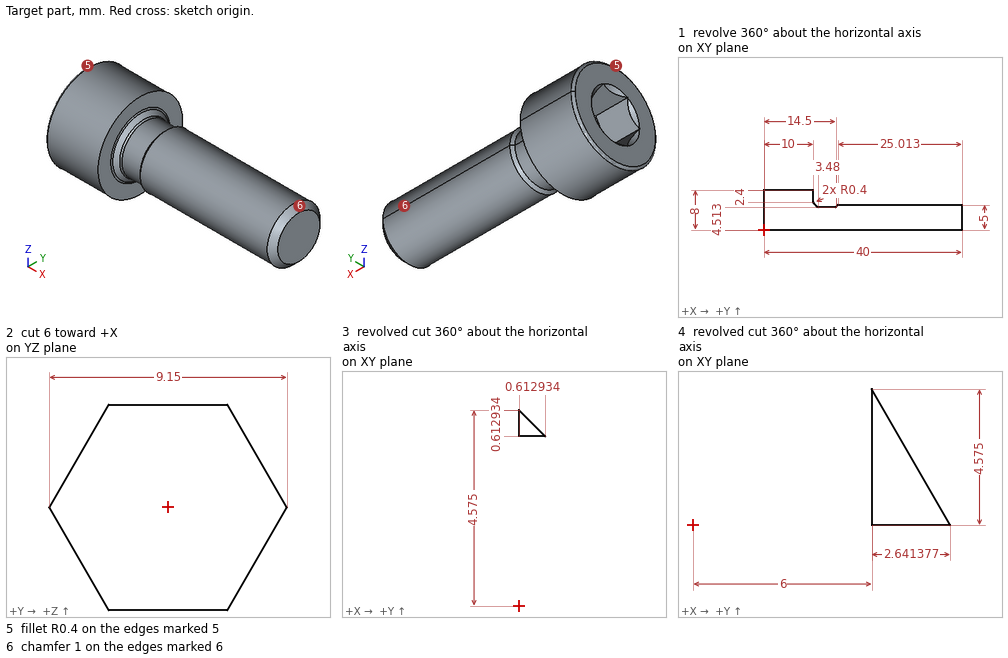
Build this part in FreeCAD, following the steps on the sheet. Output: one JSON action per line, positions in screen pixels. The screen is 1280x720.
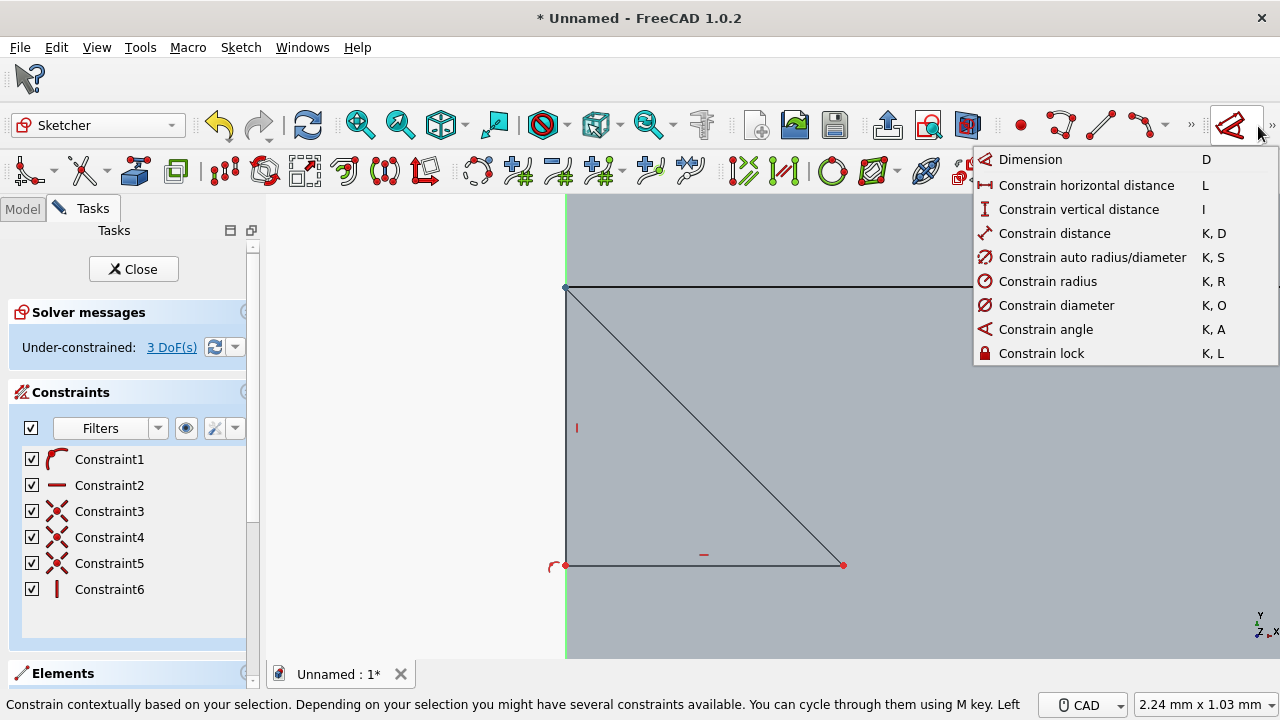
{"action": "left_click", "coordinate": [1126, 209]}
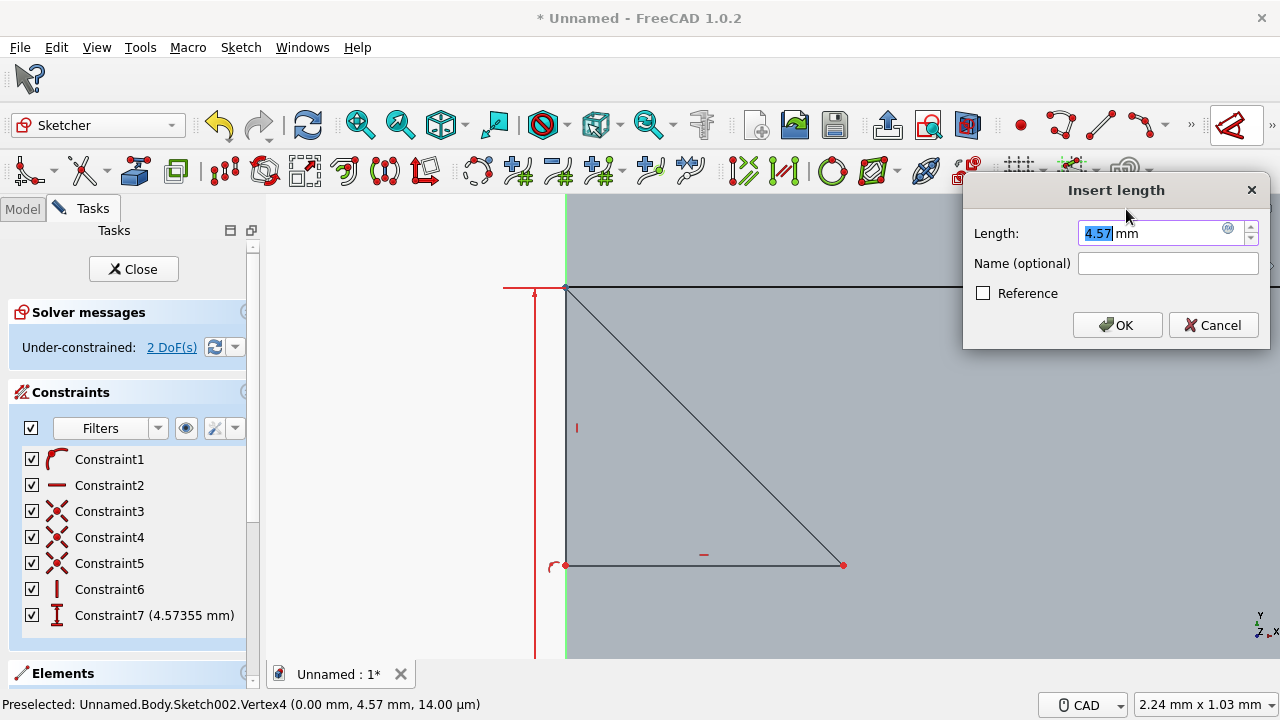
{"action": "type", "text": "4.575"}
{"action": "key", "text": "Return"}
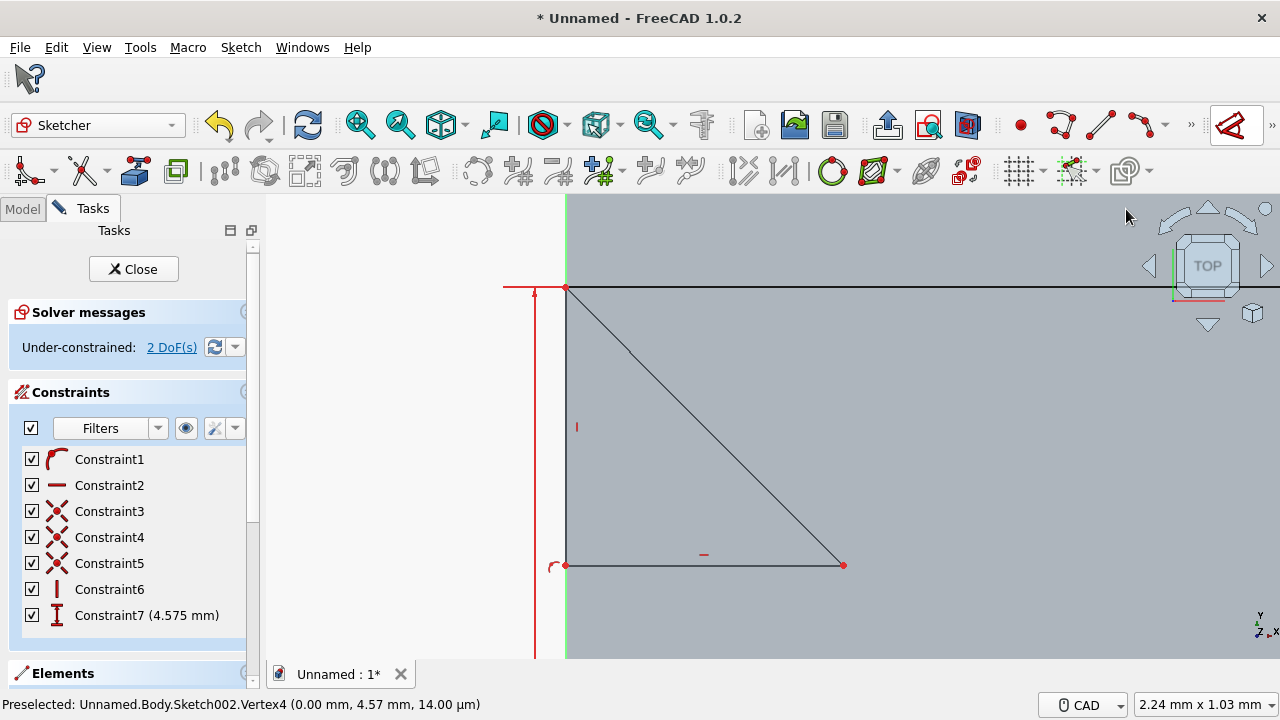
{"action": "left_click", "coordinate": [649, 566]}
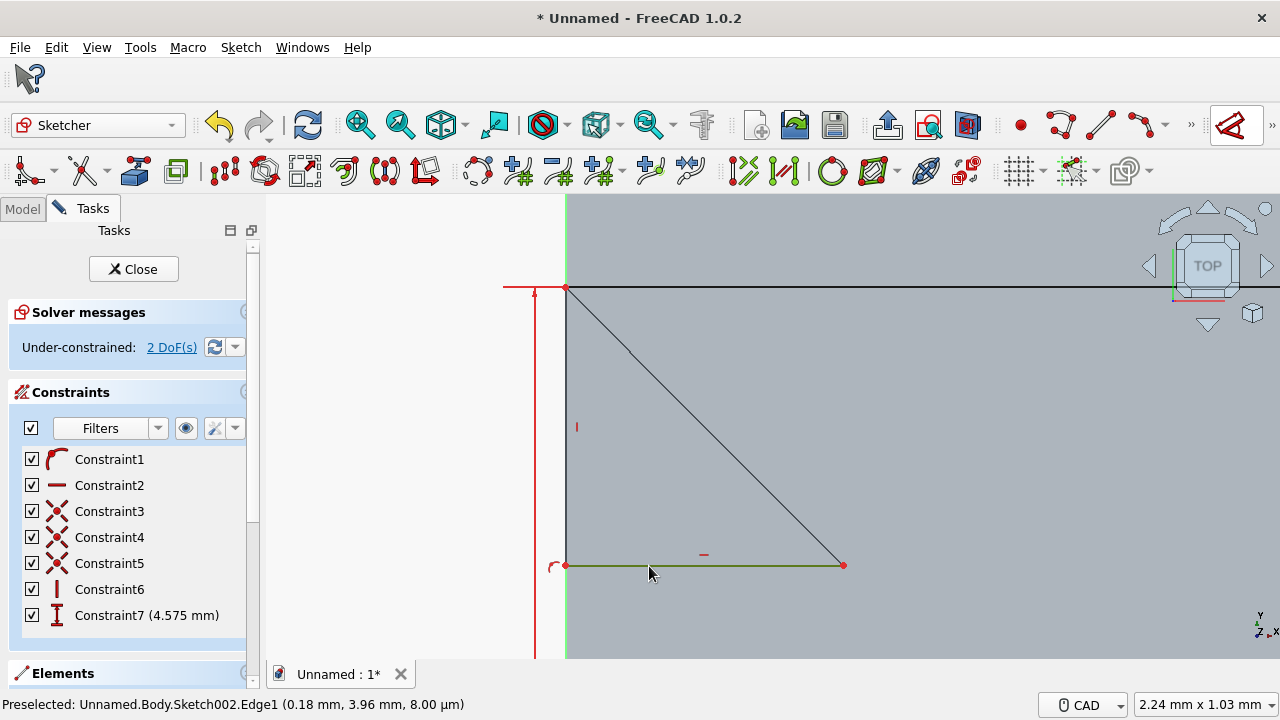
{"action": "left_click", "coordinate": [1258, 126]}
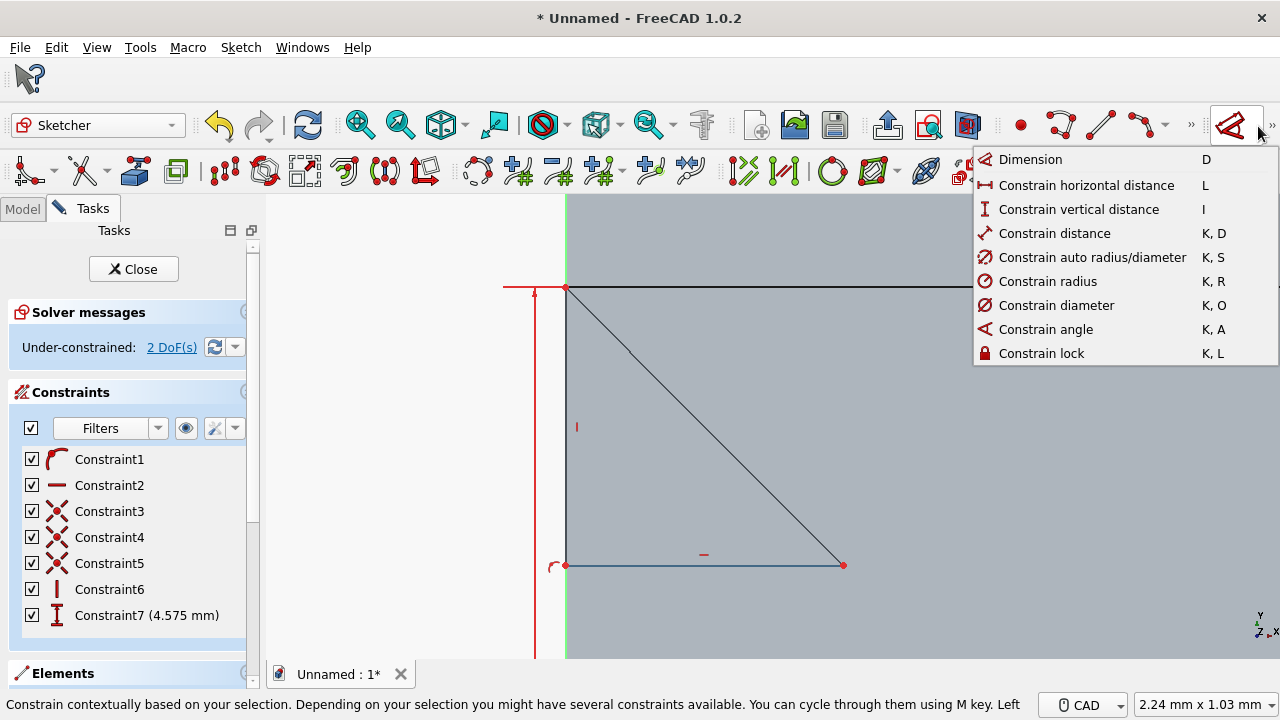
{"action": "left_click", "coordinate": [1126, 185]}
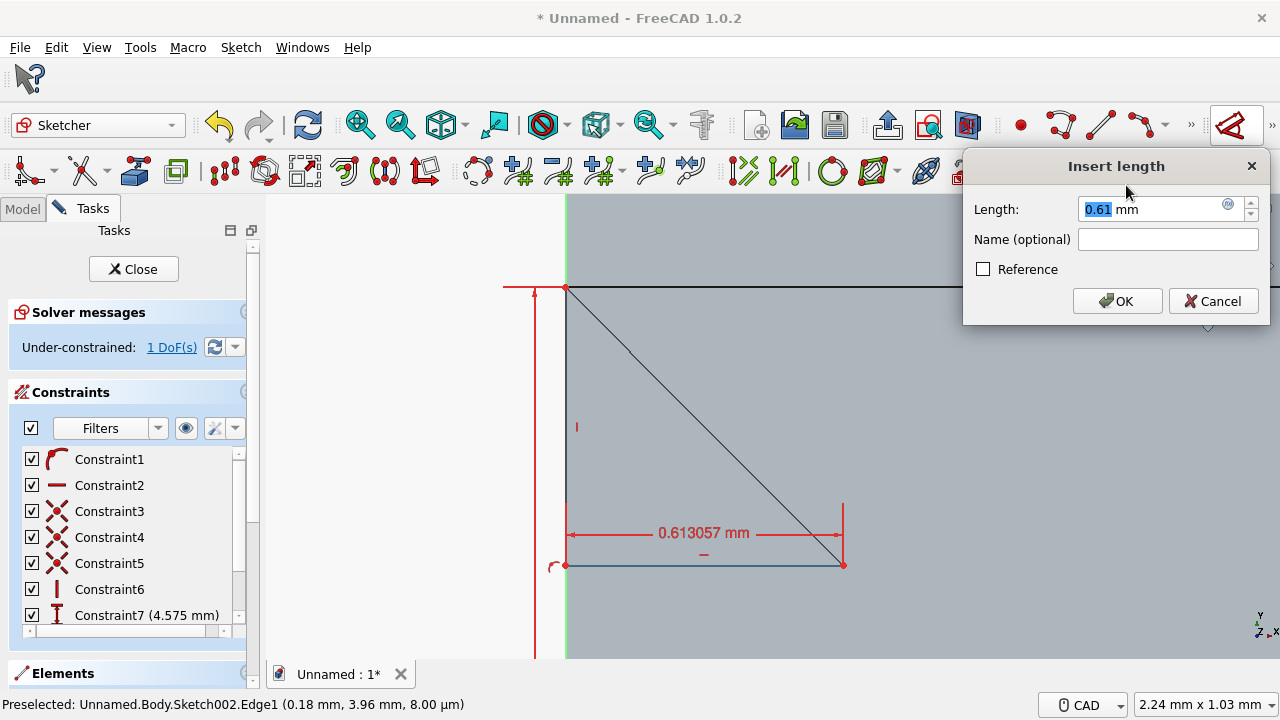
{"action": "type", "text": "0.612934"}
{"action": "key", "text": "Return"}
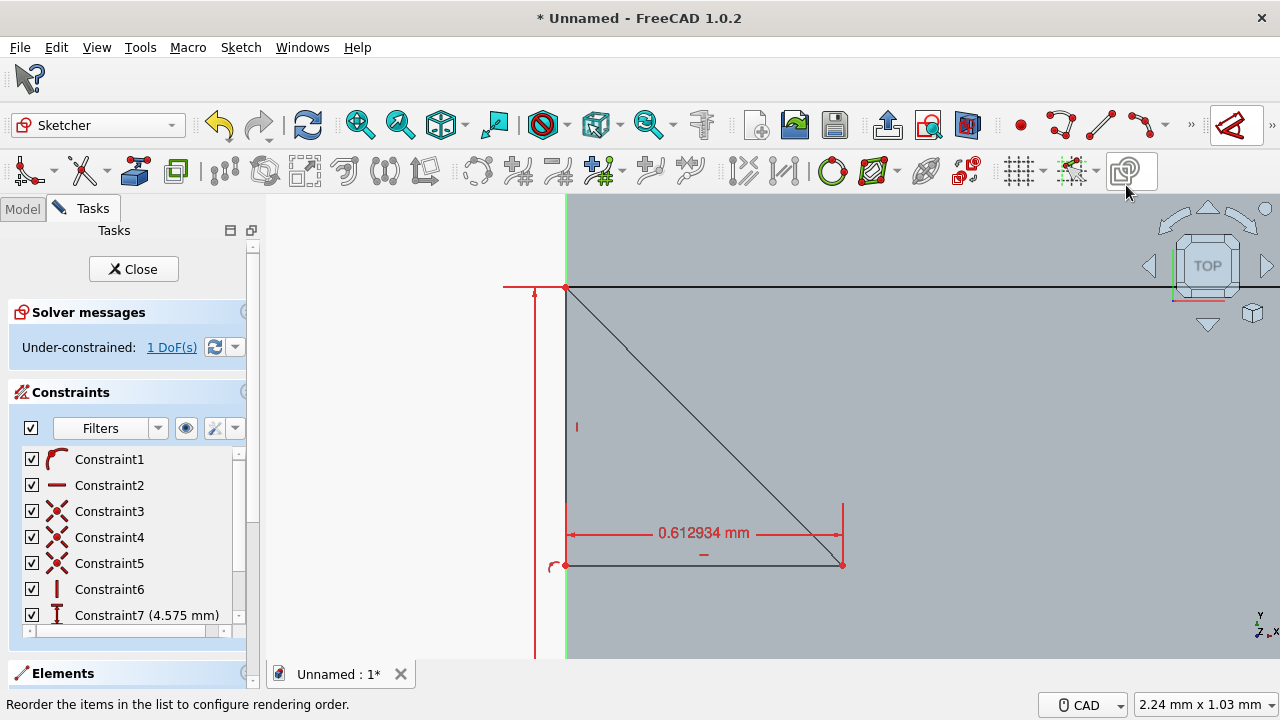
{"action": "left_click", "coordinate": [566, 371]}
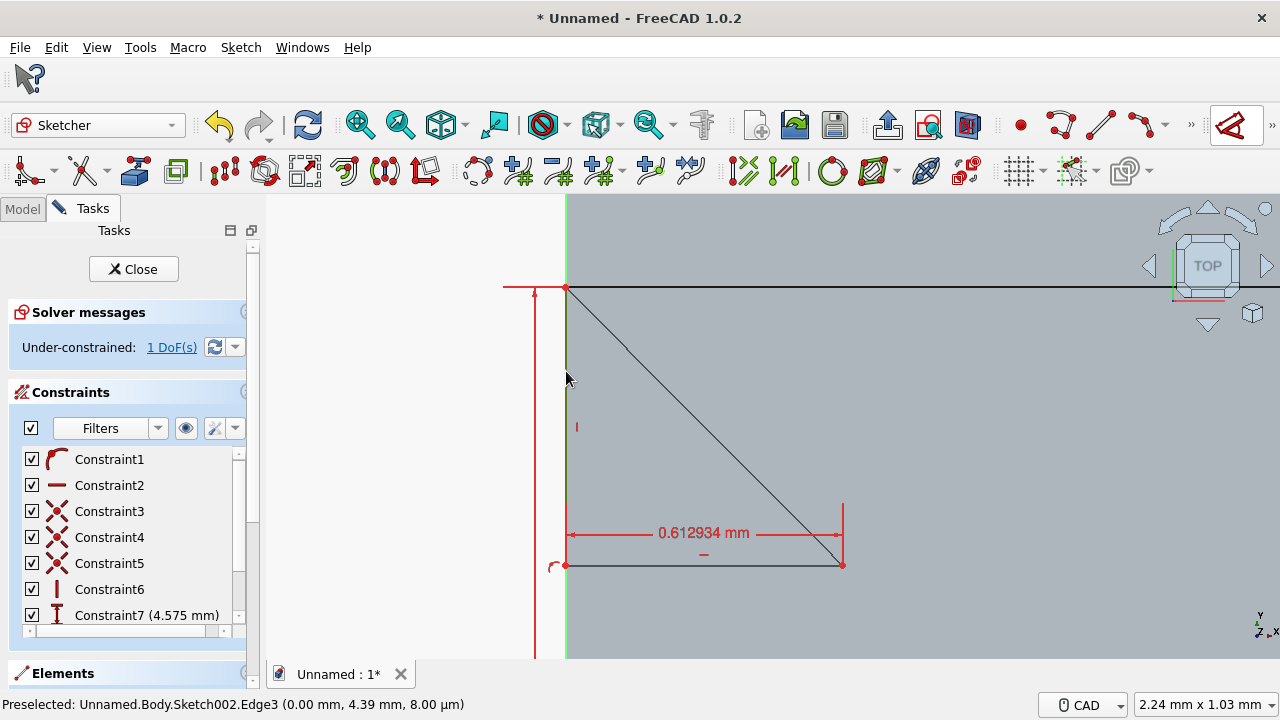
{"action": "left_click", "coordinate": [1258, 126]}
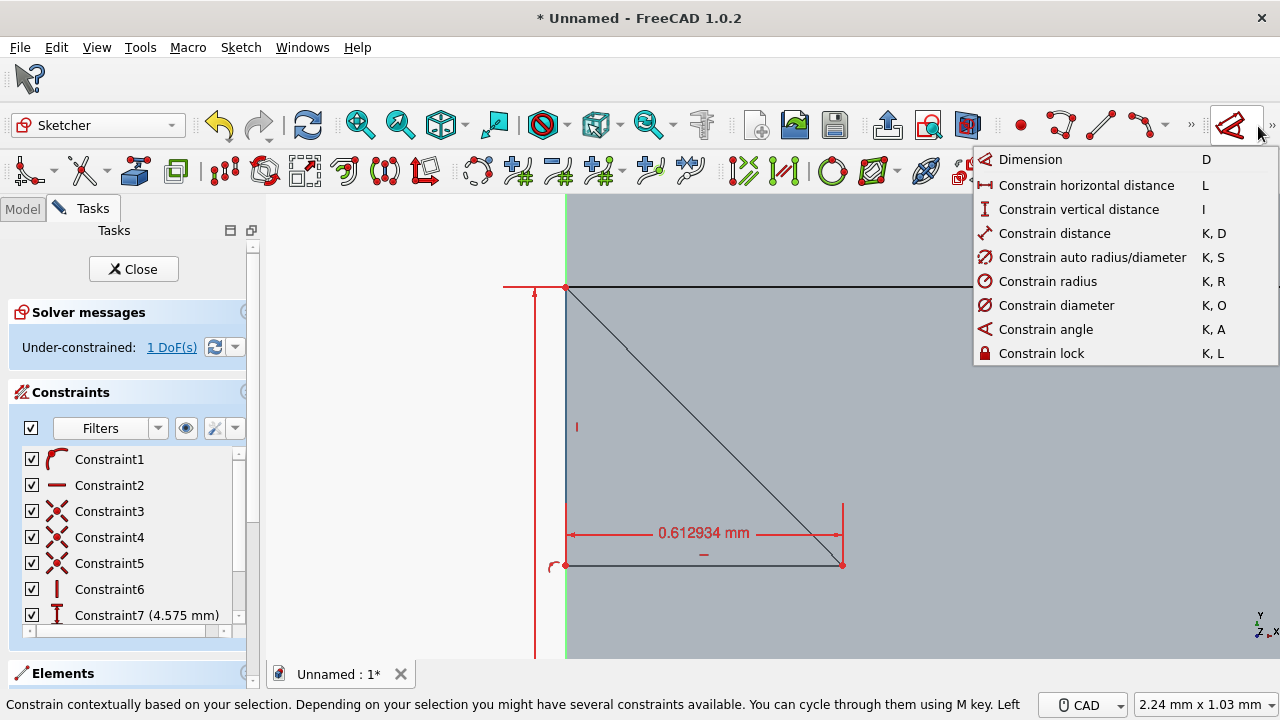
{"action": "left_click", "coordinate": [1126, 209]}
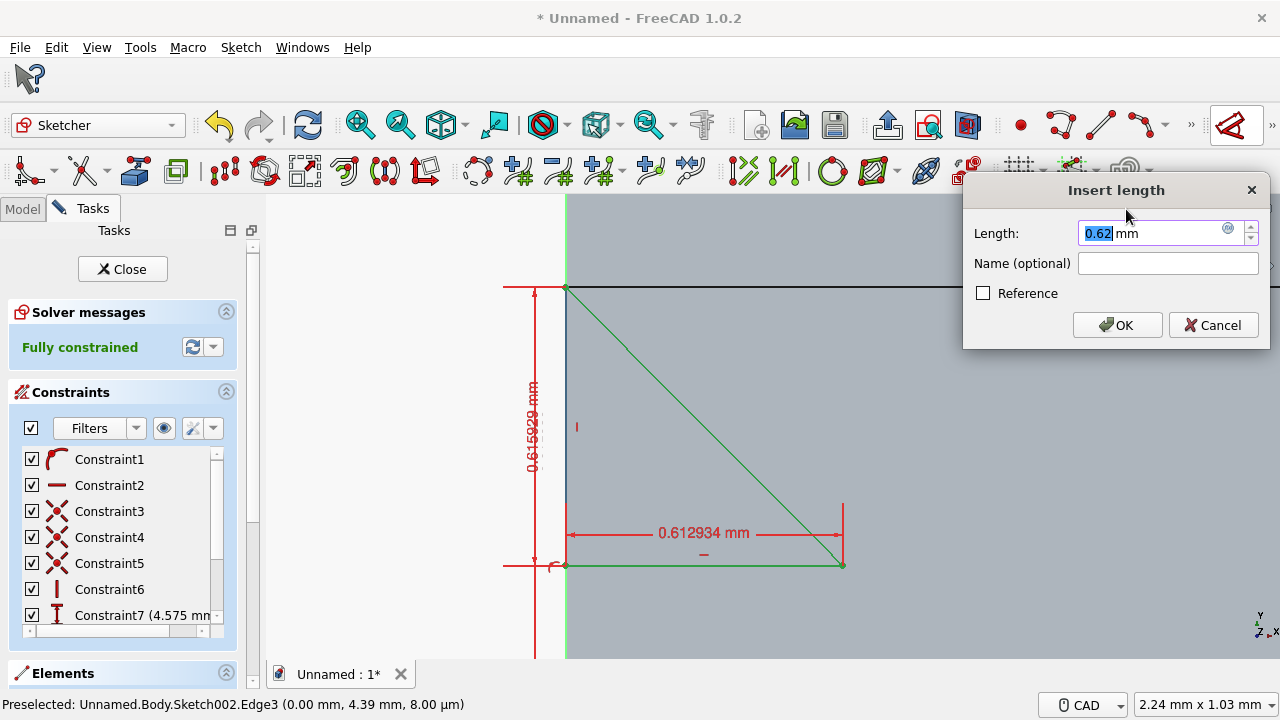
{"action": "type", "text": "0.612934"}
{"action": "key", "text": "Return"}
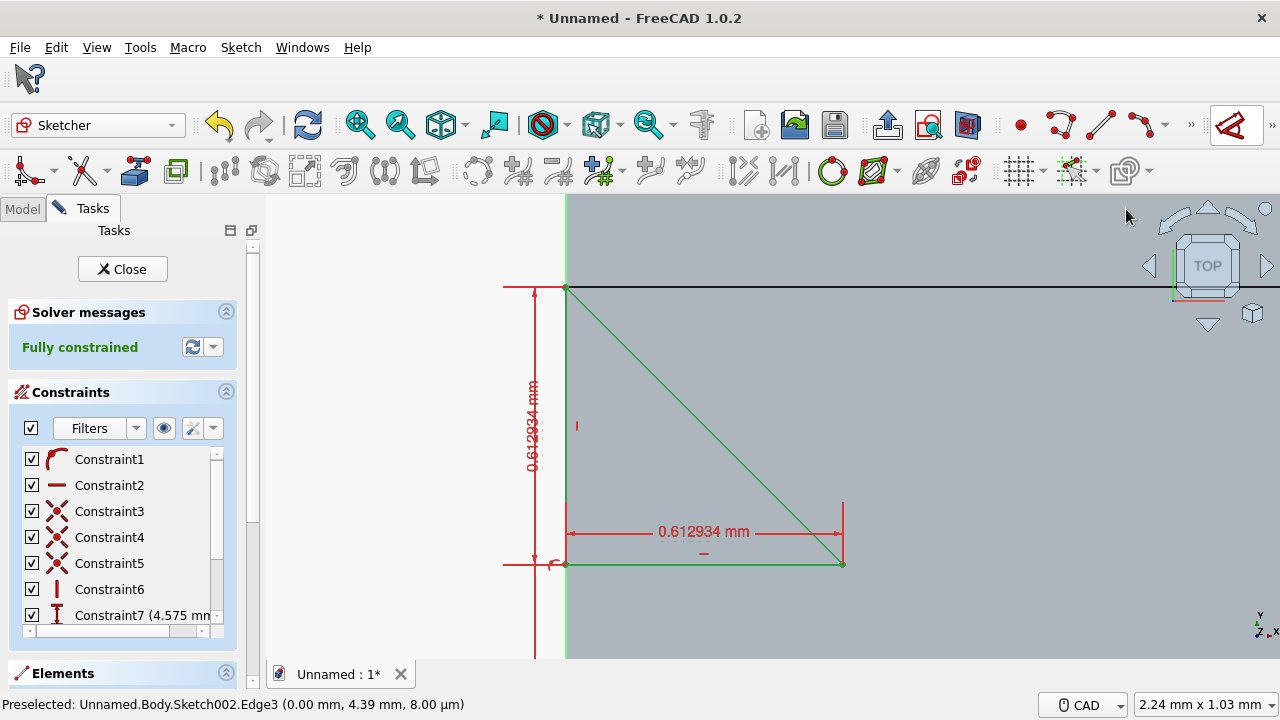
{"action": "left_click", "coordinate": [123, 269]}